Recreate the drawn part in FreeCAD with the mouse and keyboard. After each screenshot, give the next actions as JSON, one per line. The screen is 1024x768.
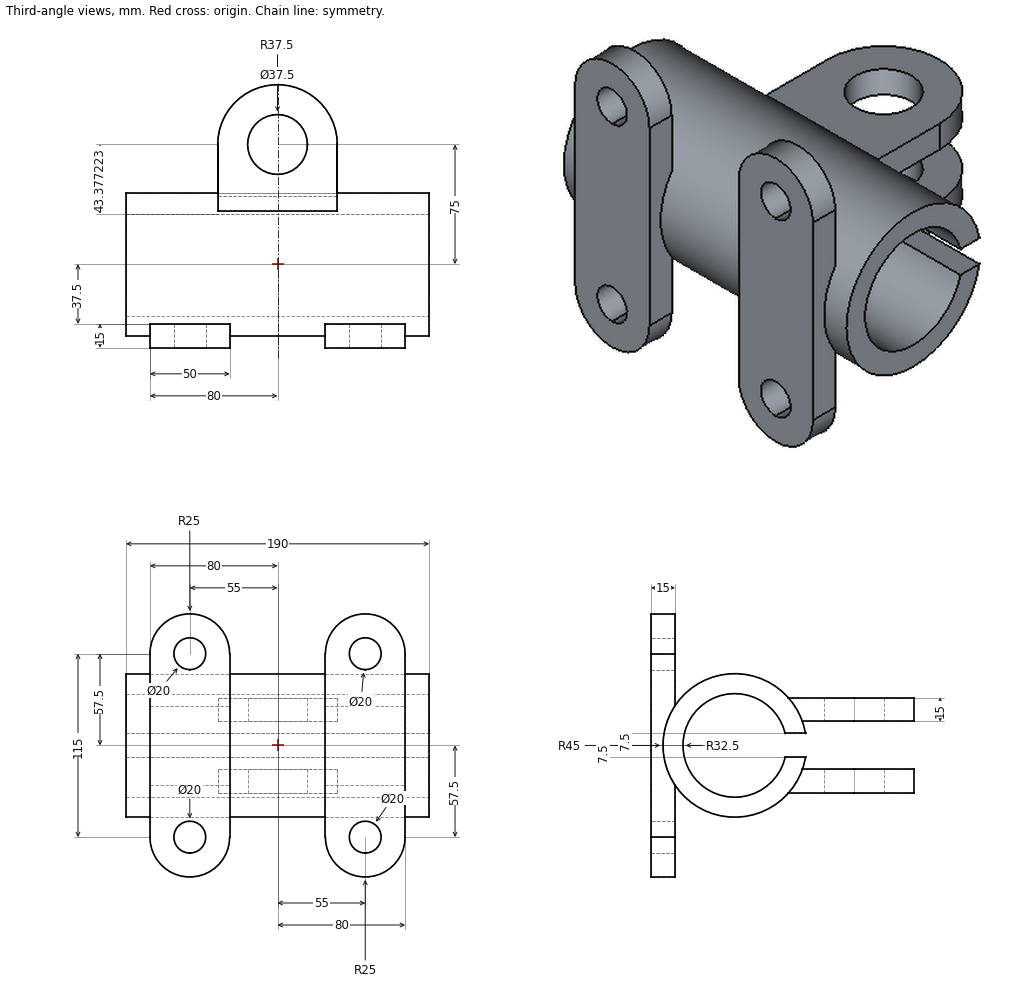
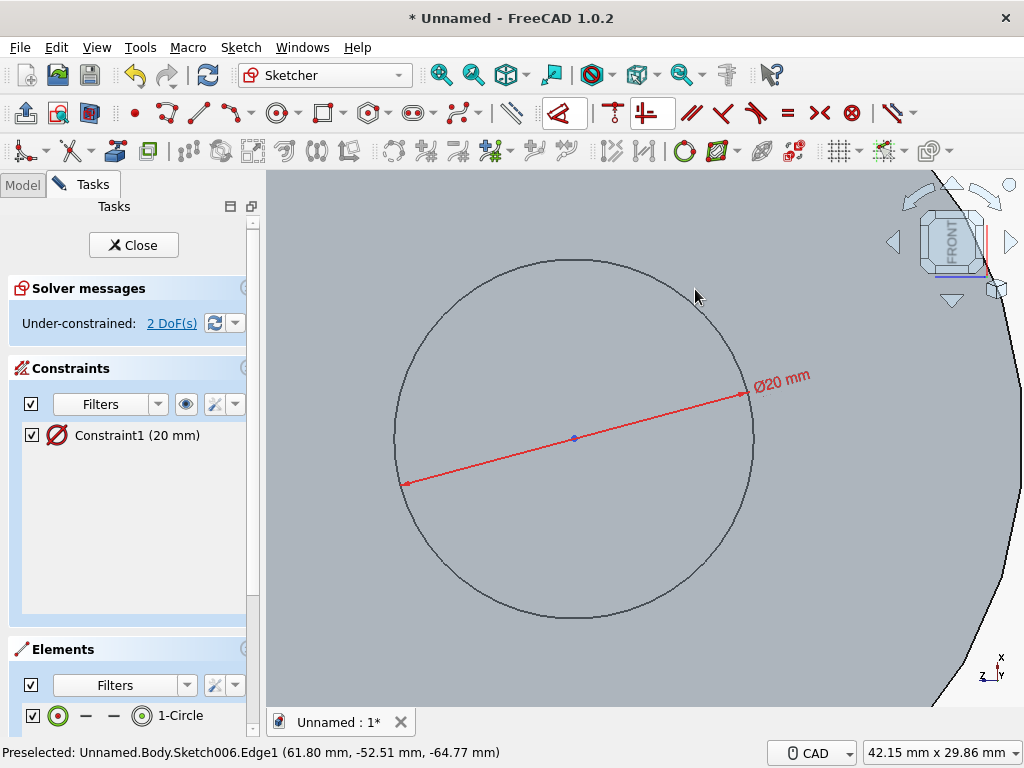
{"action": "left_click", "coordinate": [574, 439]}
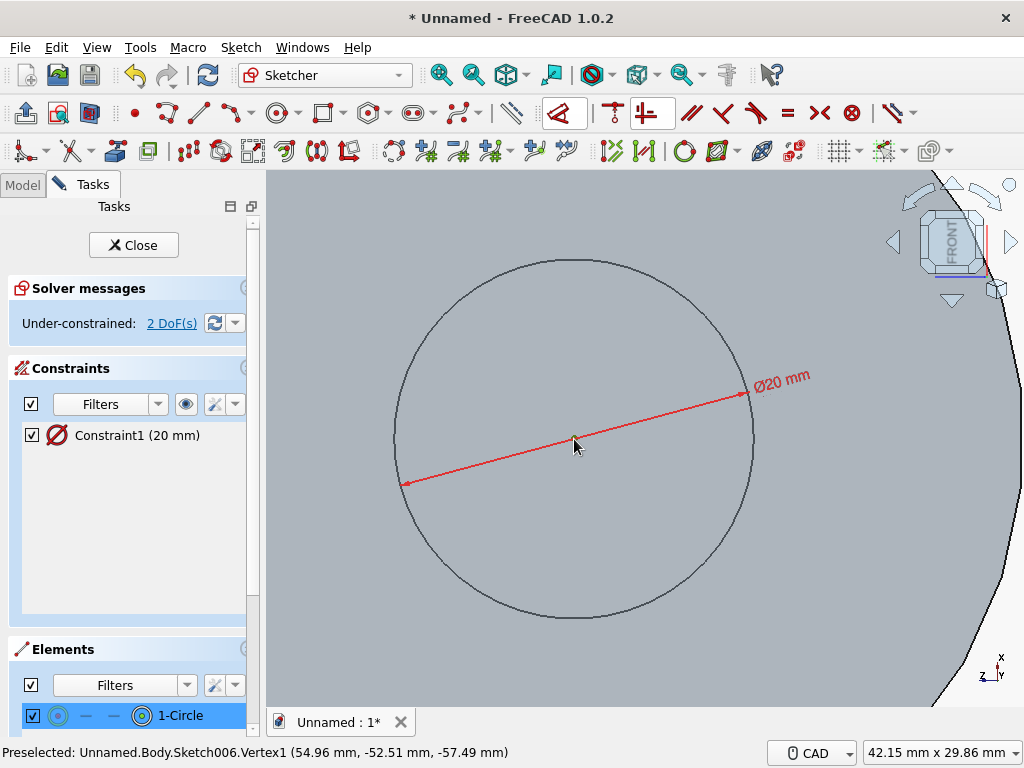
{"action": "left_click", "coordinate": [582, 114]}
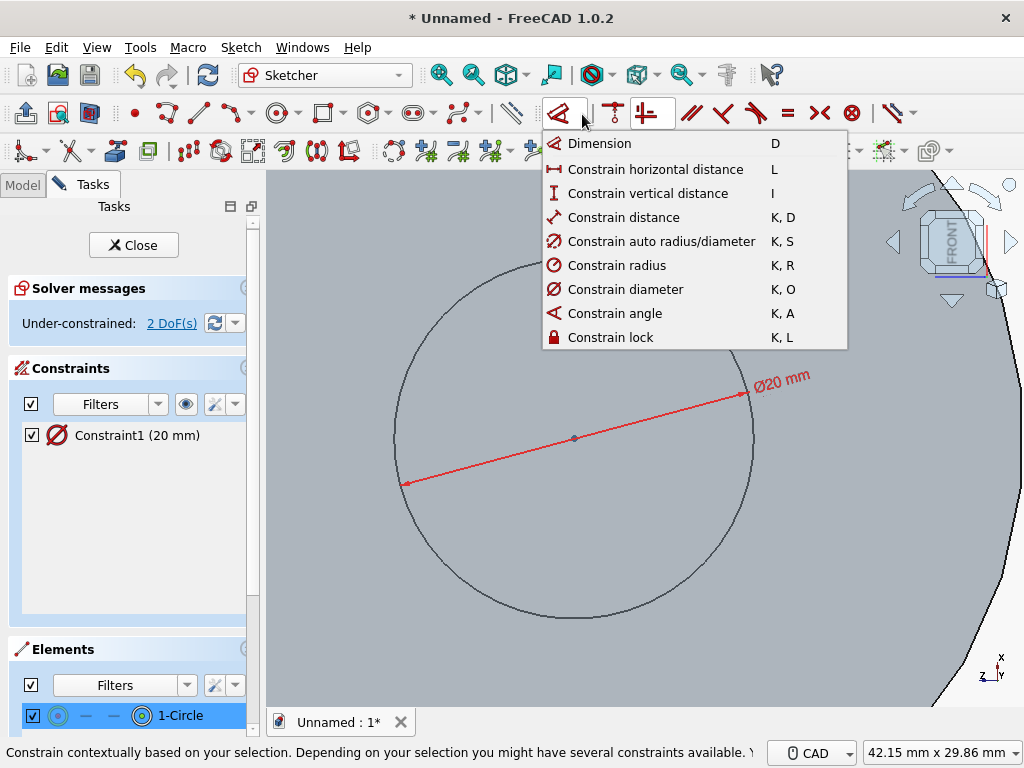
{"action": "left_click", "coordinate": [695, 193]}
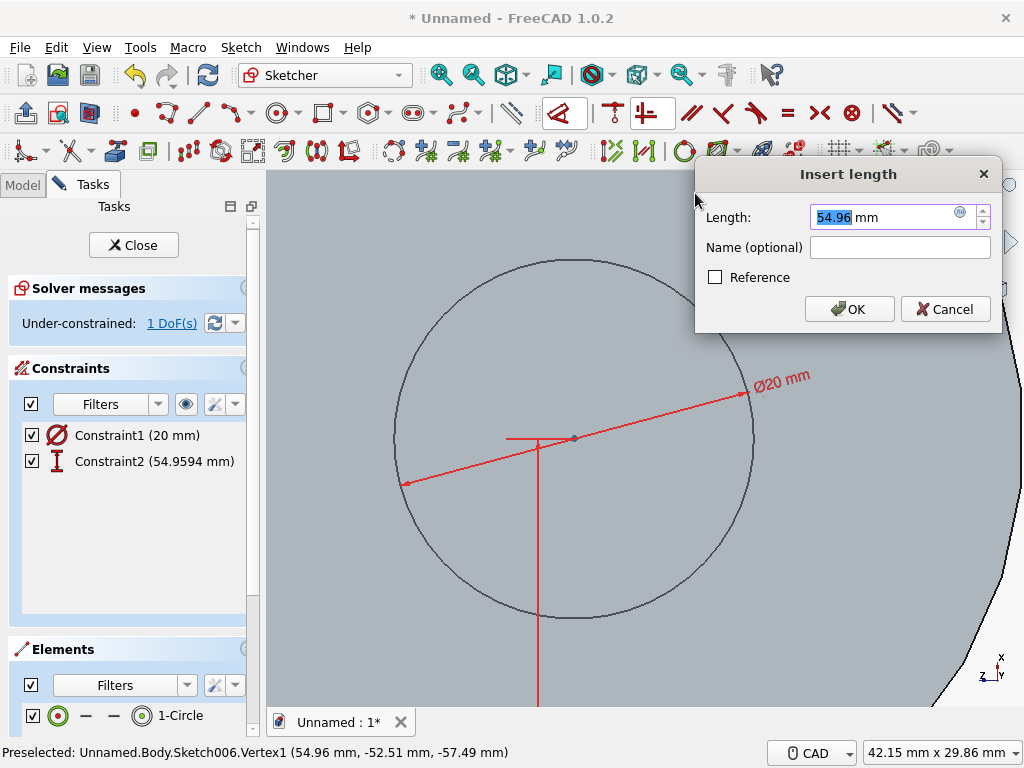
{"action": "type", "text": "55"}
{"action": "key", "text": "Return"}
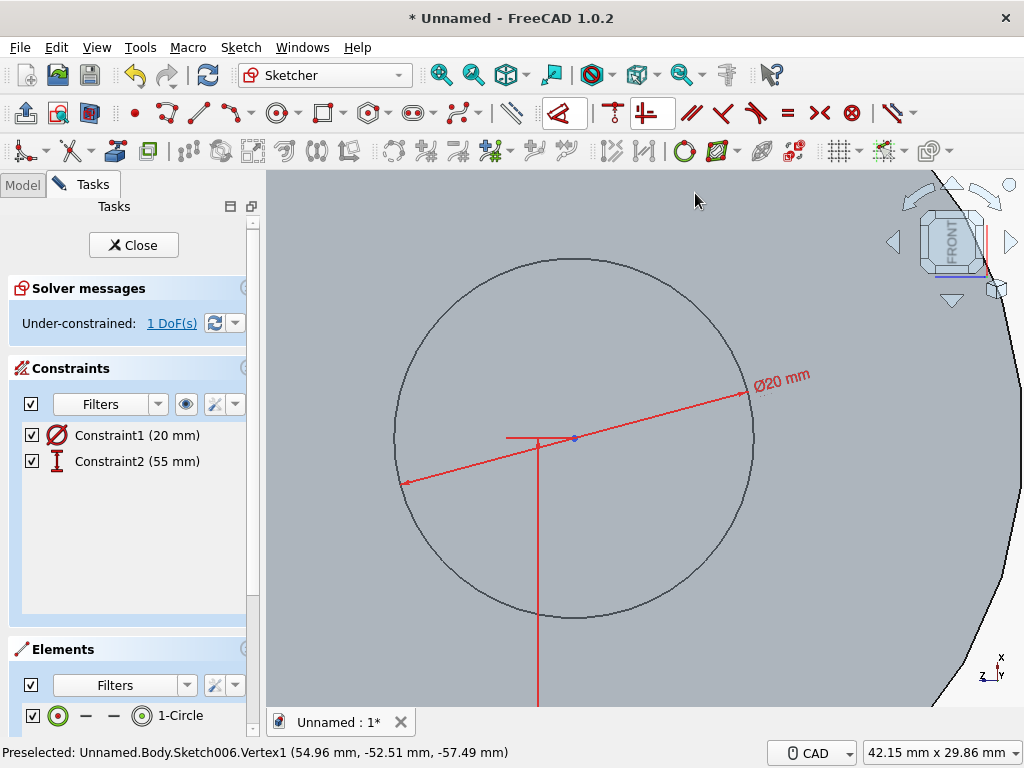
{"action": "left_click", "coordinate": [574, 438]}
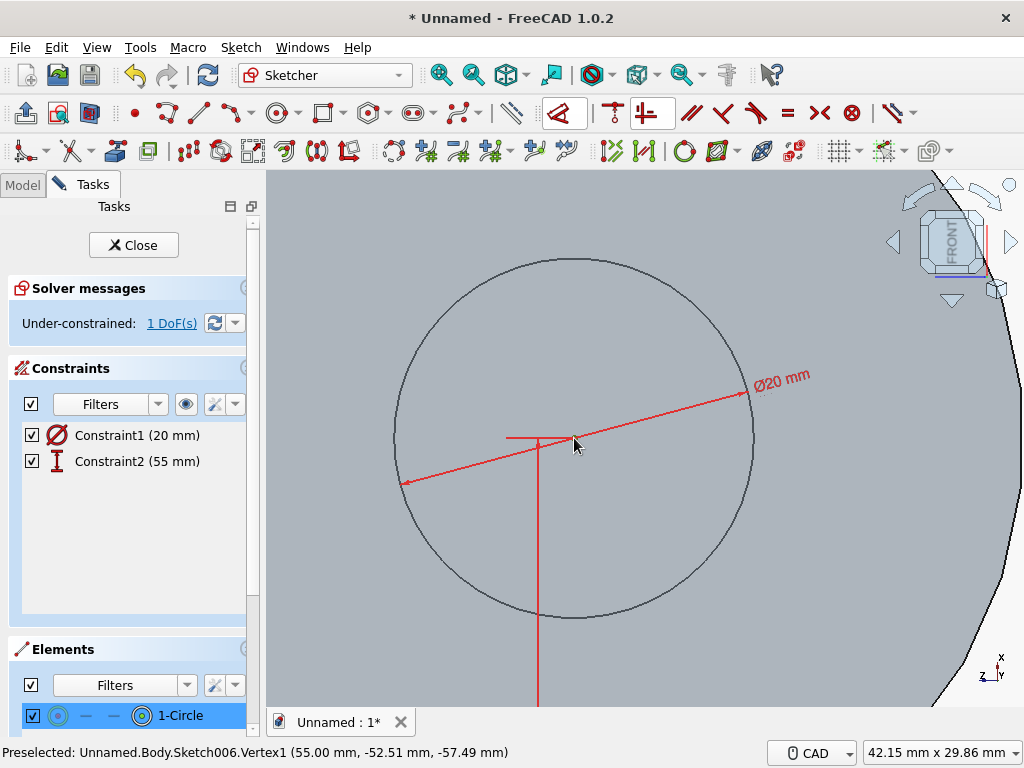
{"action": "left_click", "coordinate": [582, 114]}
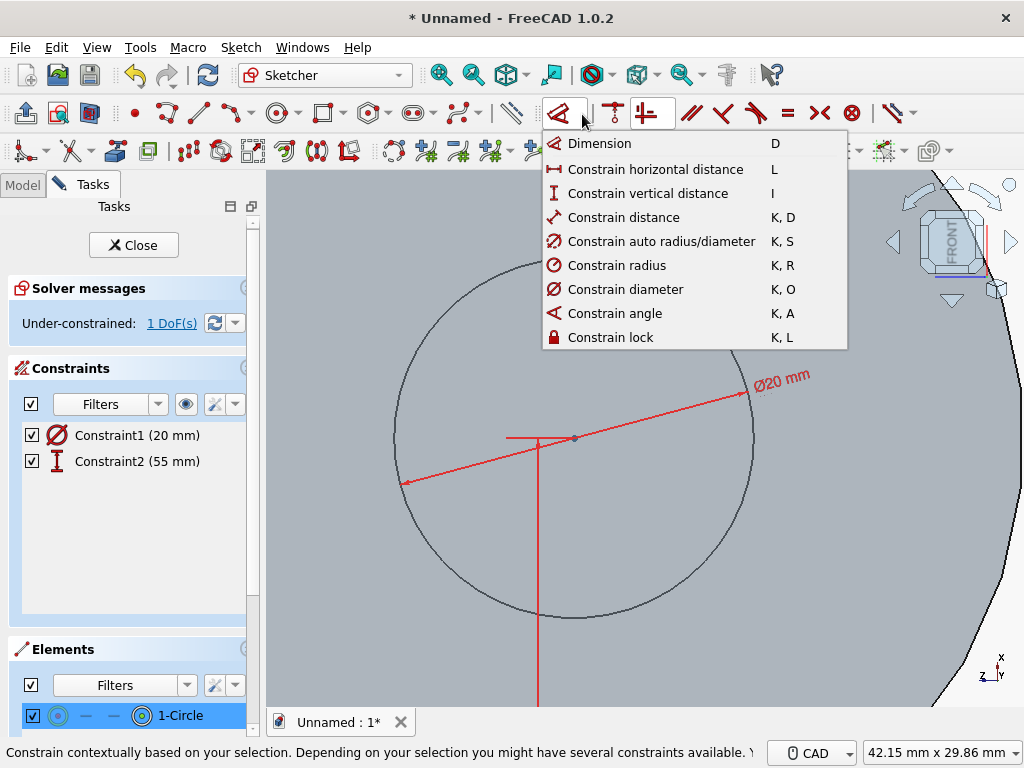
{"action": "left_click", "coordinate": [695, 169]}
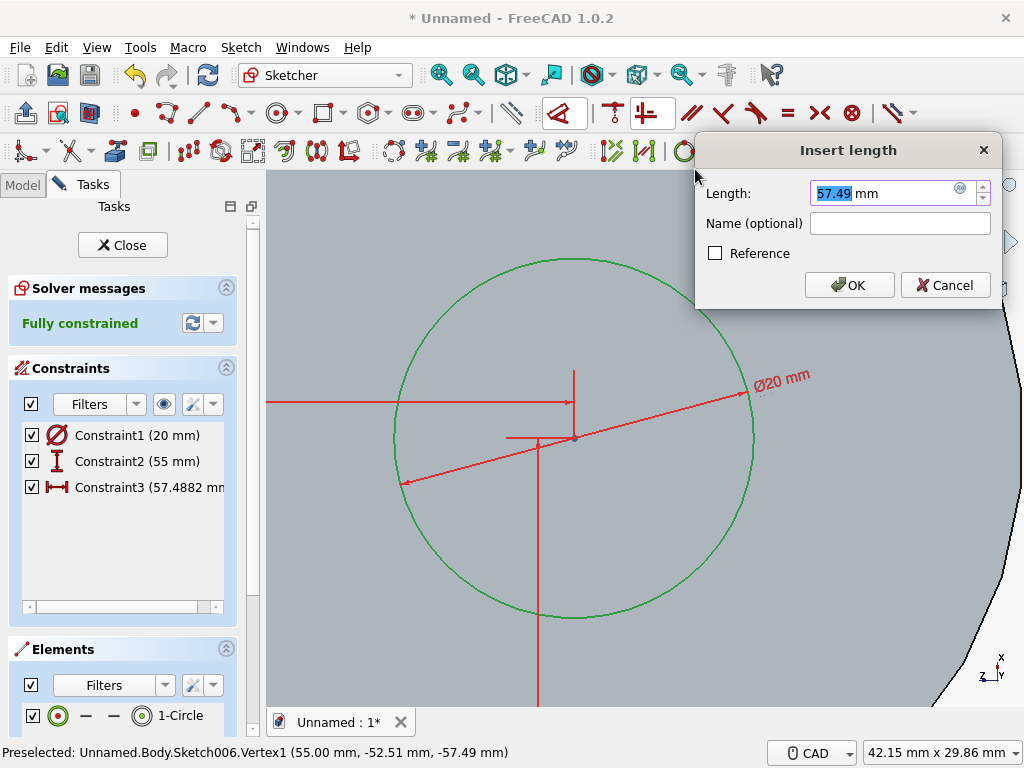
{"action": "type", "text": "57.5"}
{"action": "key", "text": "Return"}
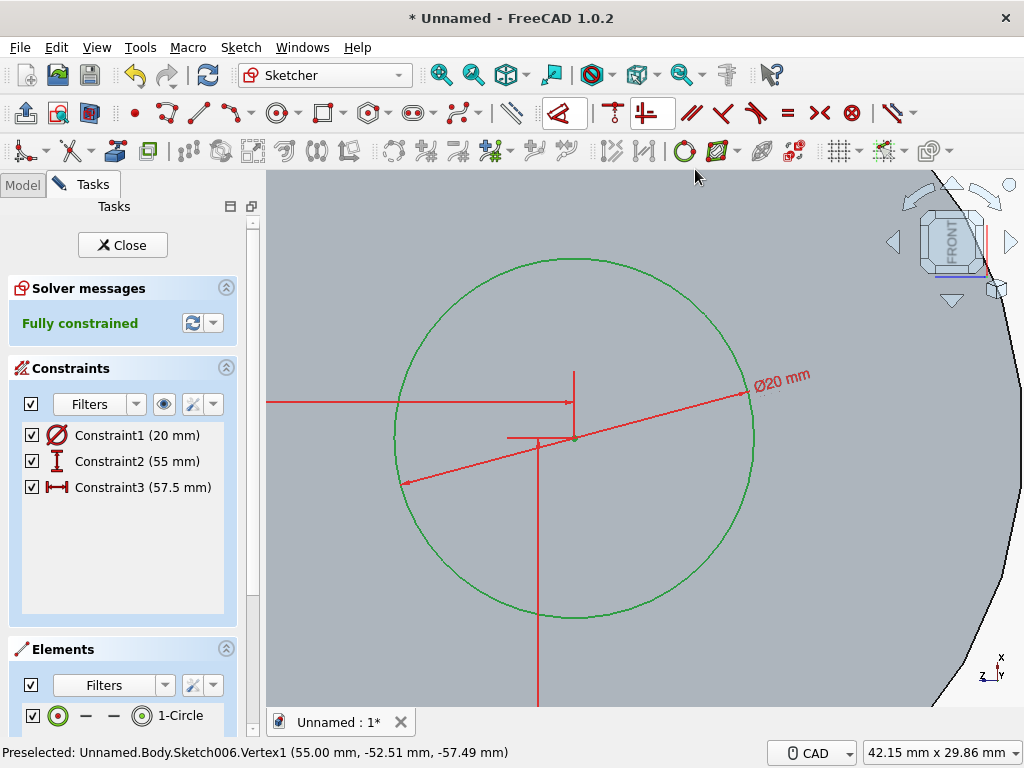
{"action": "left_click", "coordinate": [123, 245]}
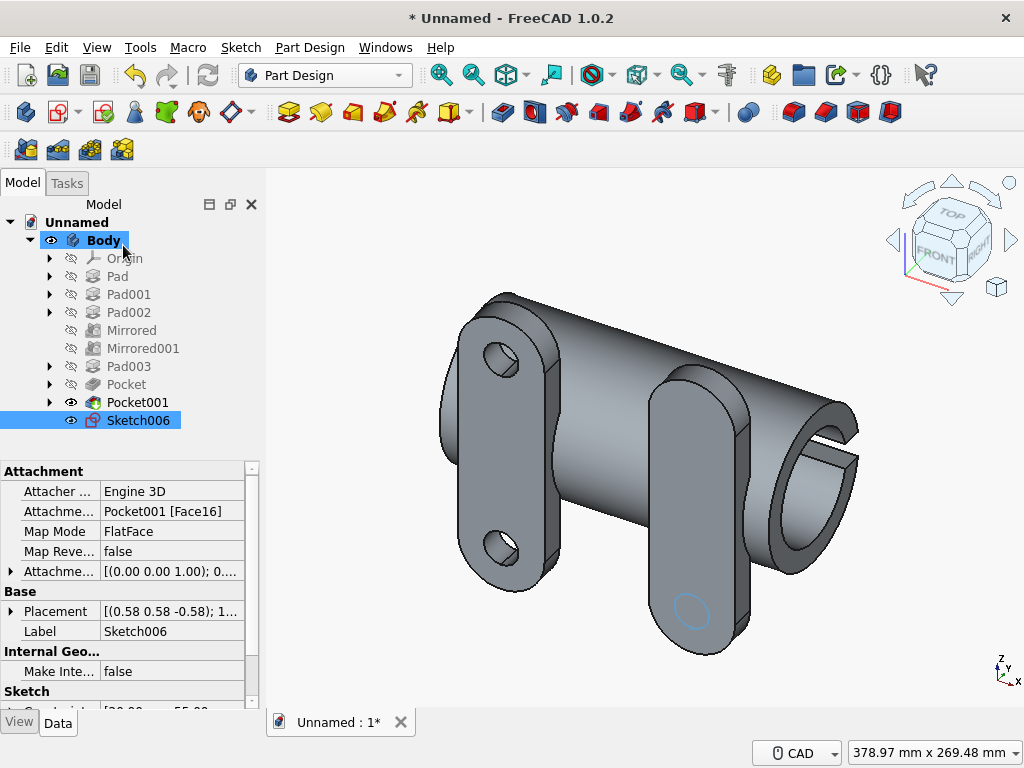
{"action": "left_click", "coordinate": [504, 112]}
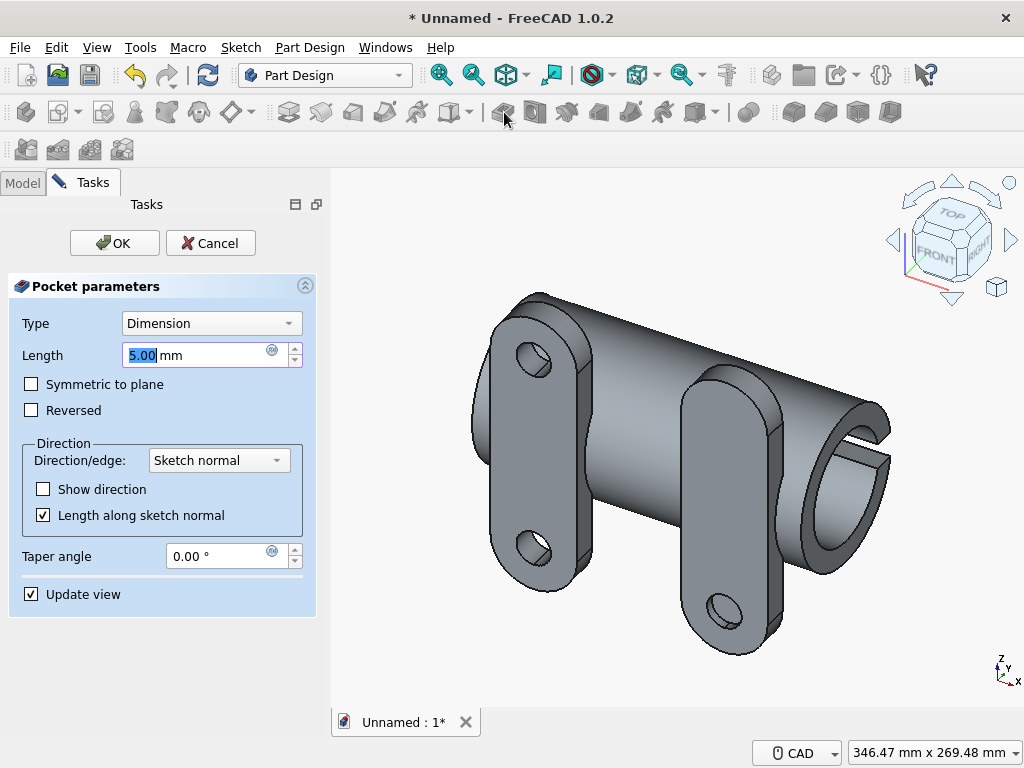
{"action": "left_click", "coordinate": [212, 324]}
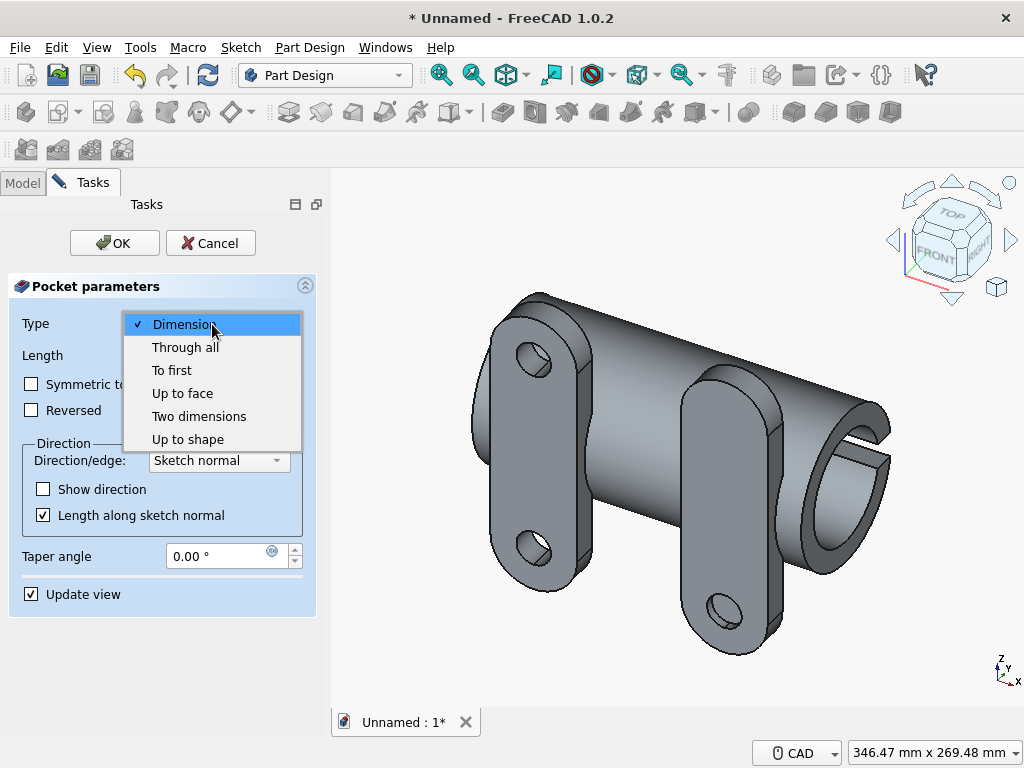
{"action": "left_click", "coordinate": [212, 370]}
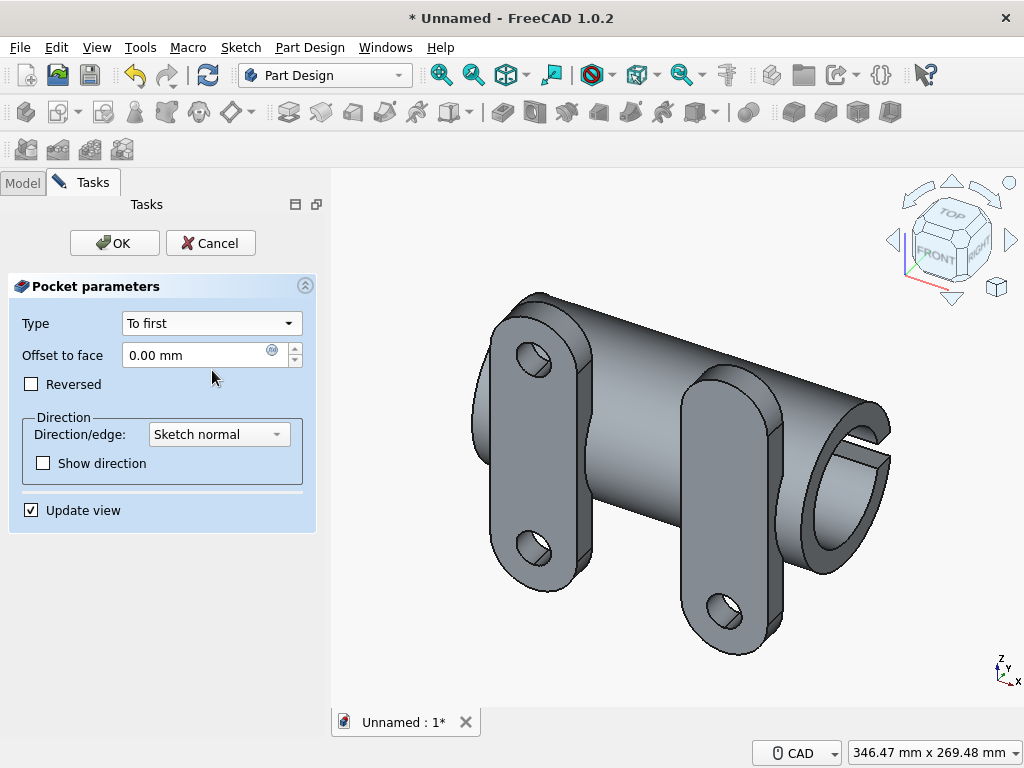
{"action": "left_click", "coordinate": [115, 243]}